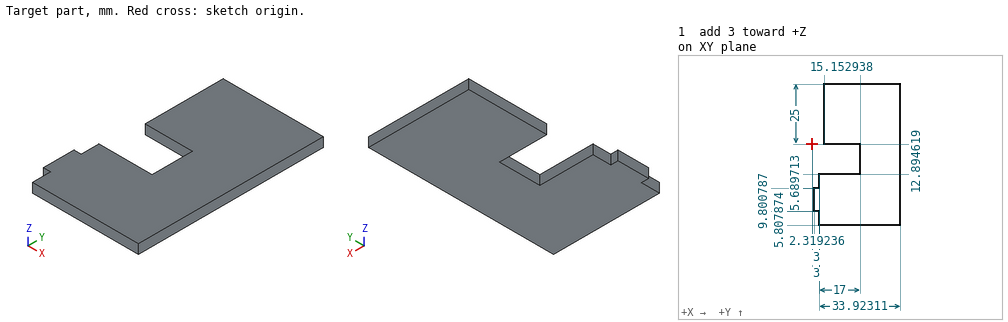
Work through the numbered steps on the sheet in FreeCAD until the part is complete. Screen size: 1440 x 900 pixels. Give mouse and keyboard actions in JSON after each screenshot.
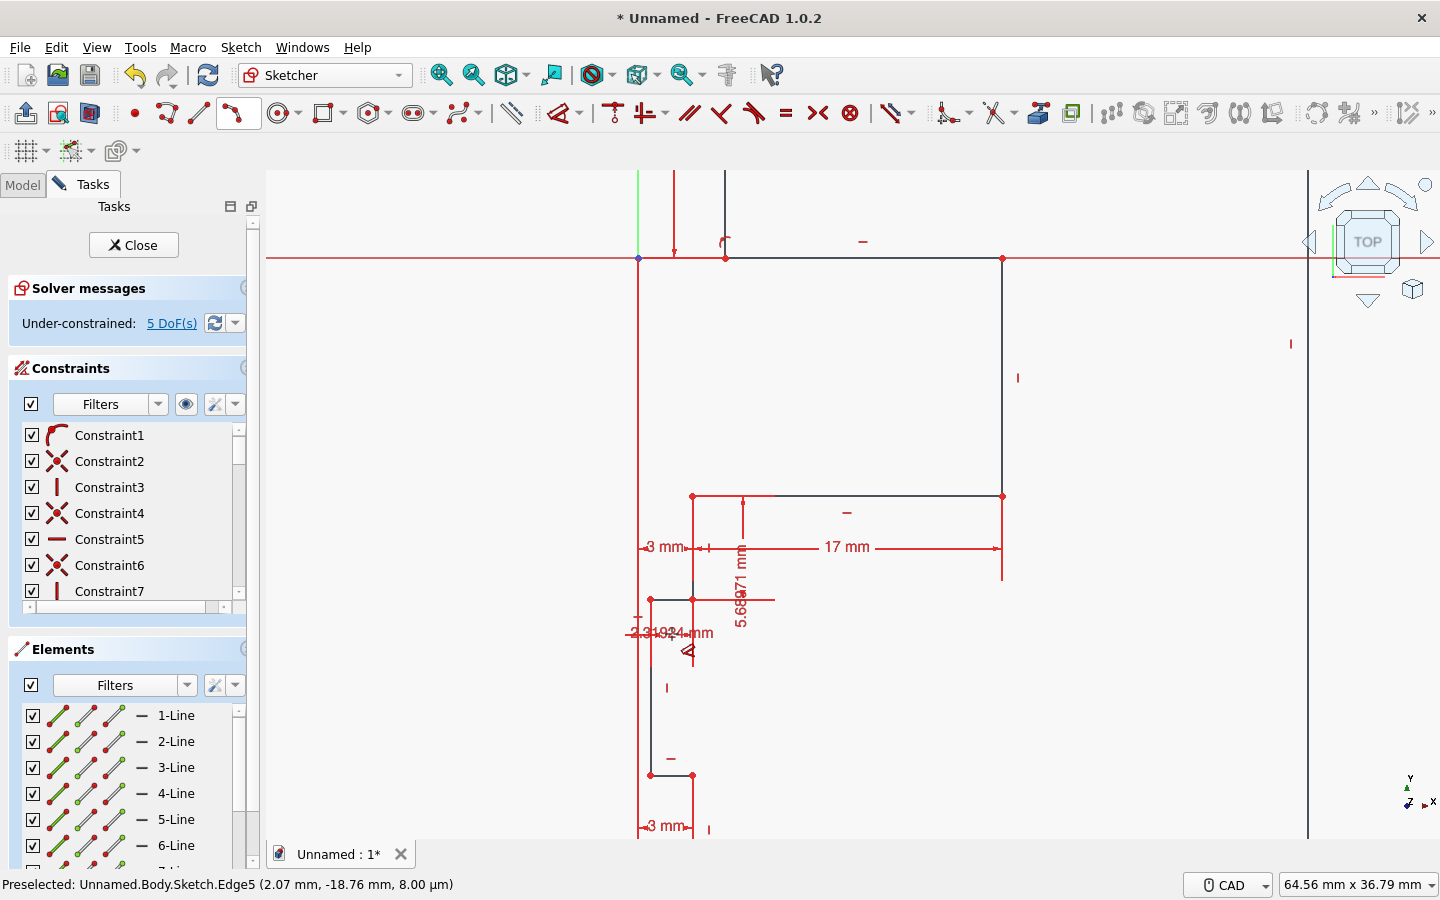
{"action": "left_click", "coordinate": [651, 652]}
{"action": "left_click", "coordinate": [617, 688]}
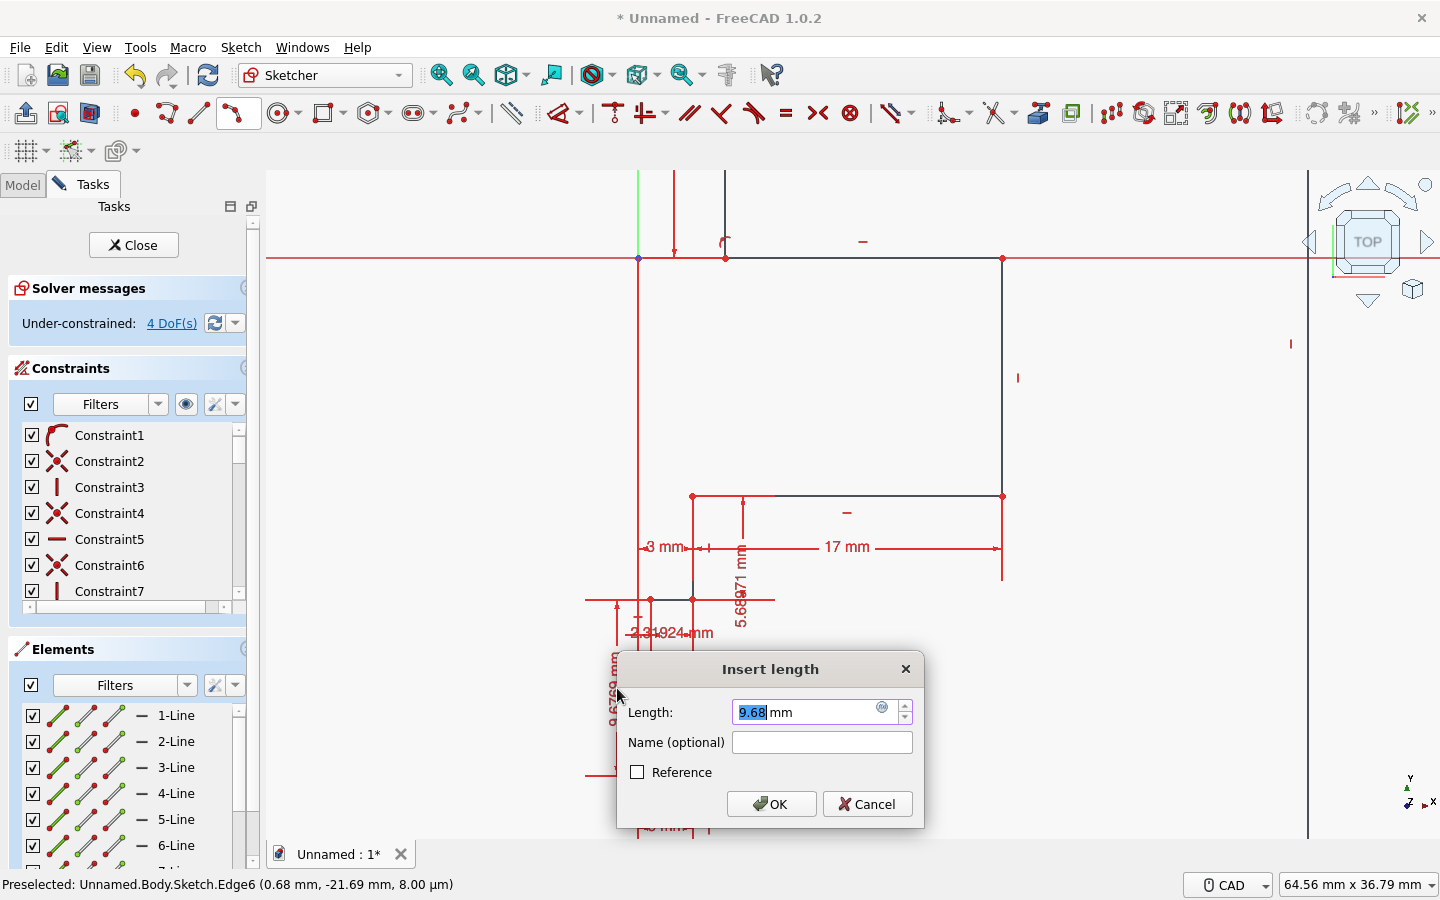
{"action": "type", "text": "9.800787"}
{"action": "key", "text": "Return"}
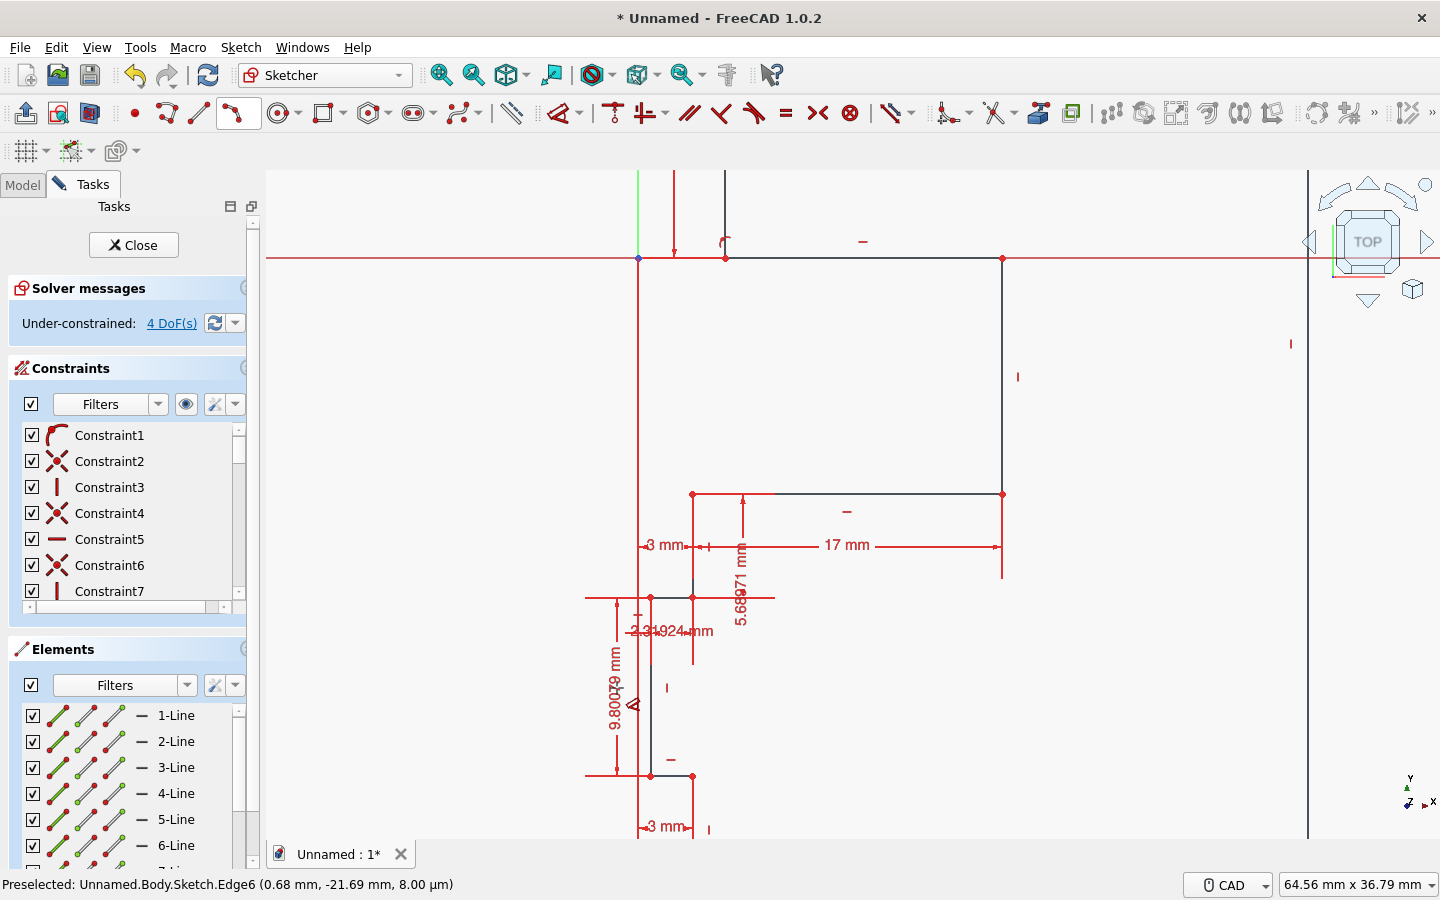
{"action": "left_click", "coordinate": [693, 808]}
{"action": "left_click", "coordinate": [659, 794]}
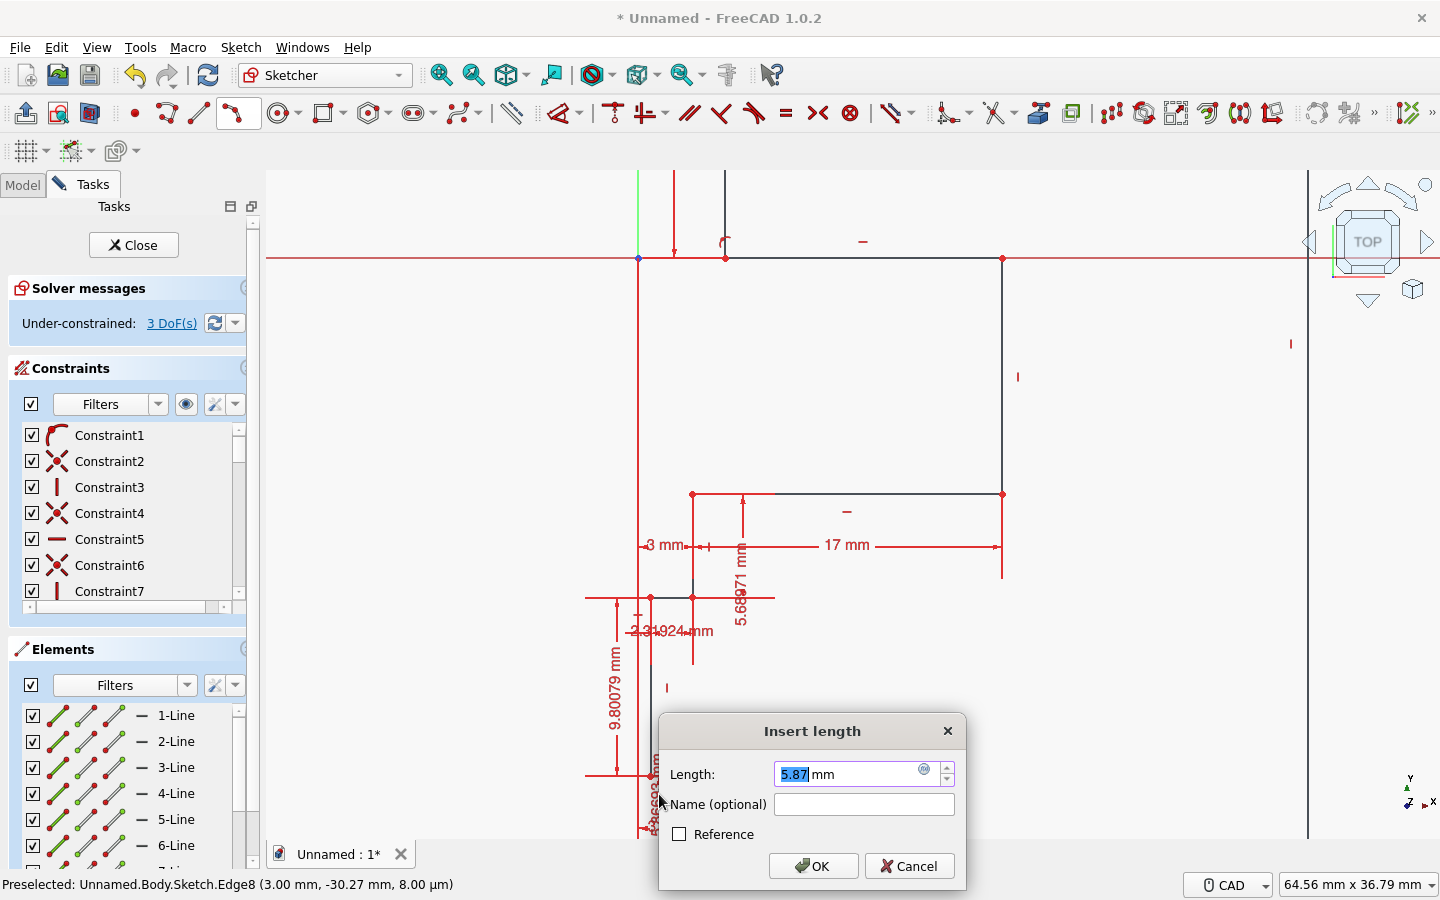
{"action": "type", "text": "5.807874"}
{"action": "key", "text": "Return"}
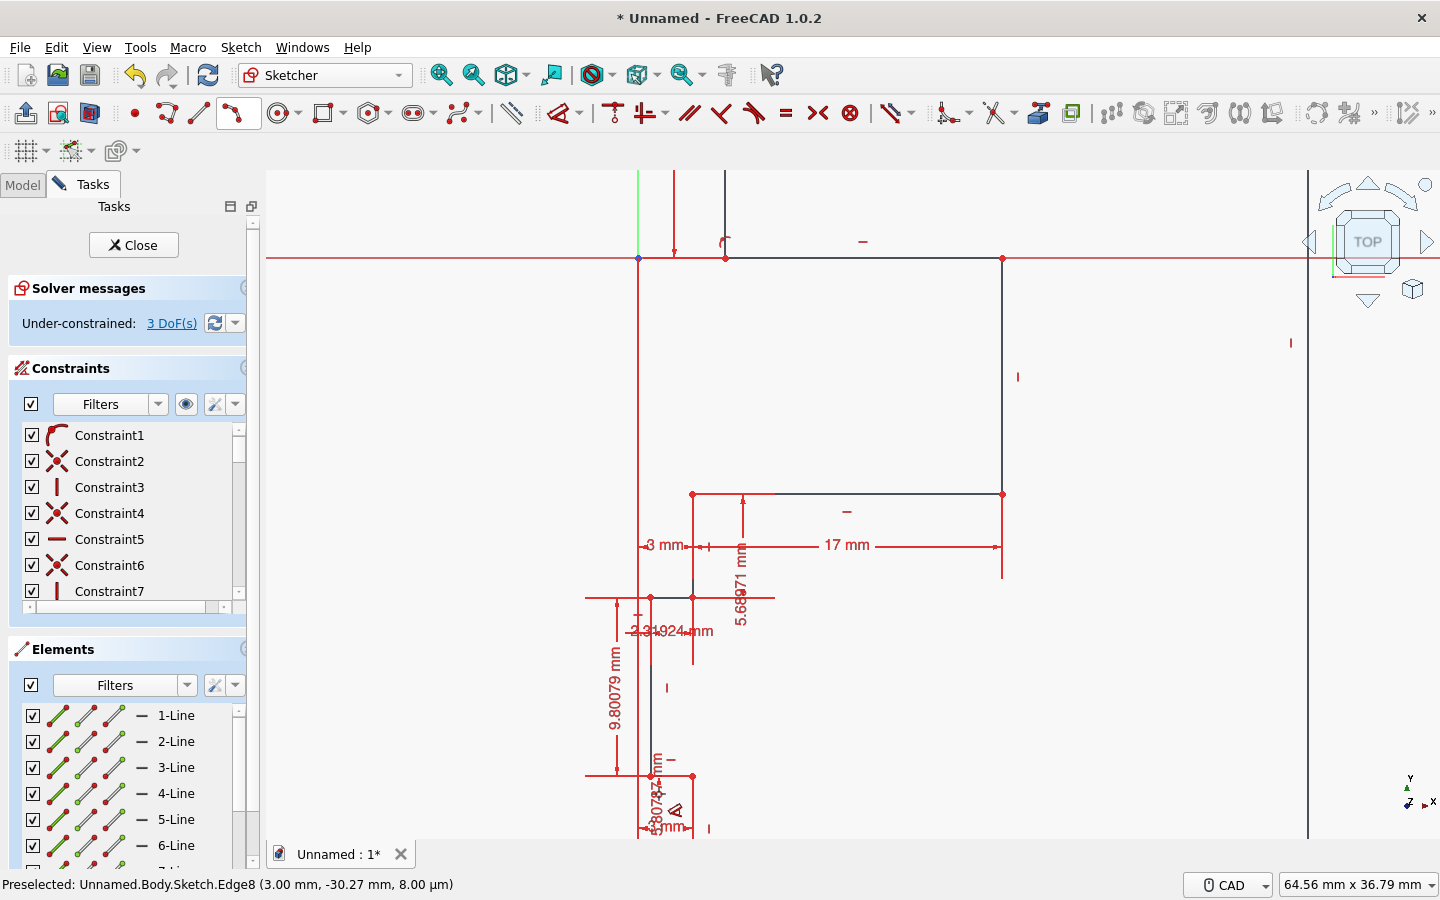
{"action": "scroll", "coordinate": [674, 599], "scroll_direction": "down", "scroll_amount": 5}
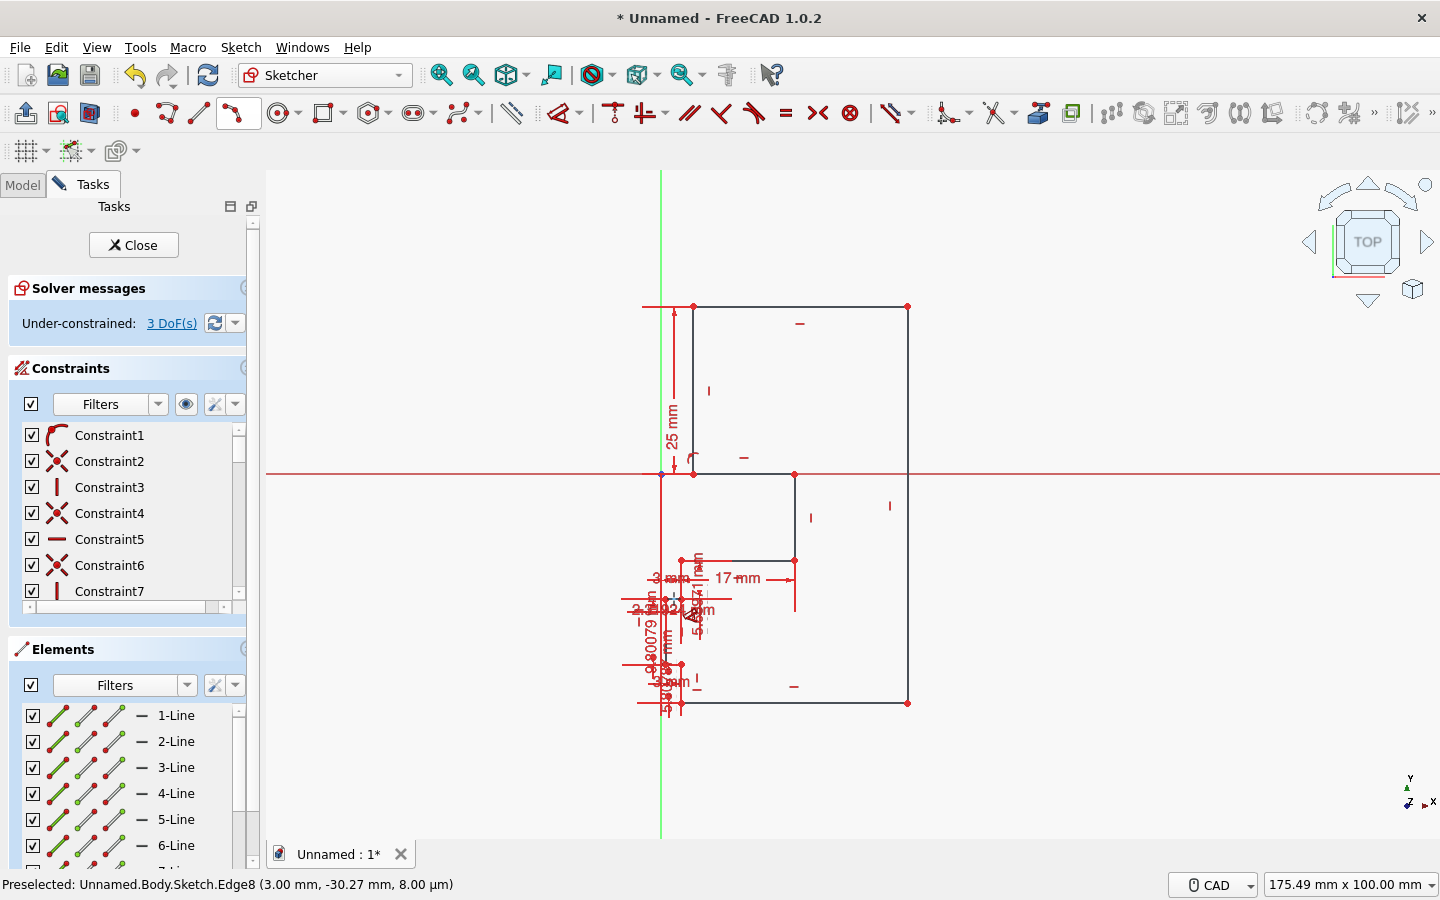
{"action": "left_click", "coordinate": [749, 703]}
{"action": "left_click", "coordinate": [794, 737]}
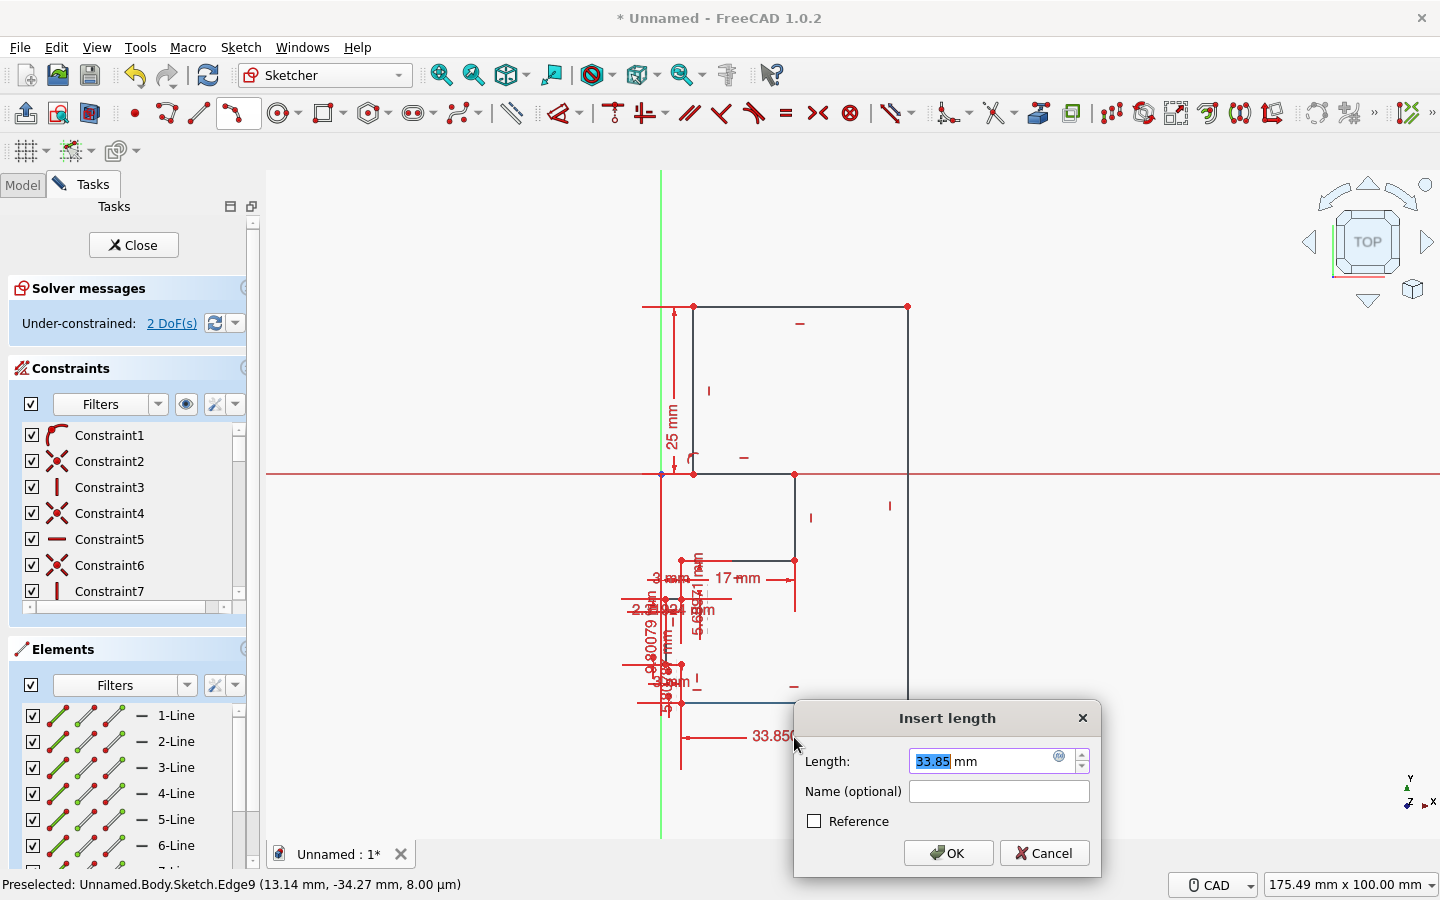
{"action": "type", "text": "33.92311"}
{"action": "key", "text": "Return"}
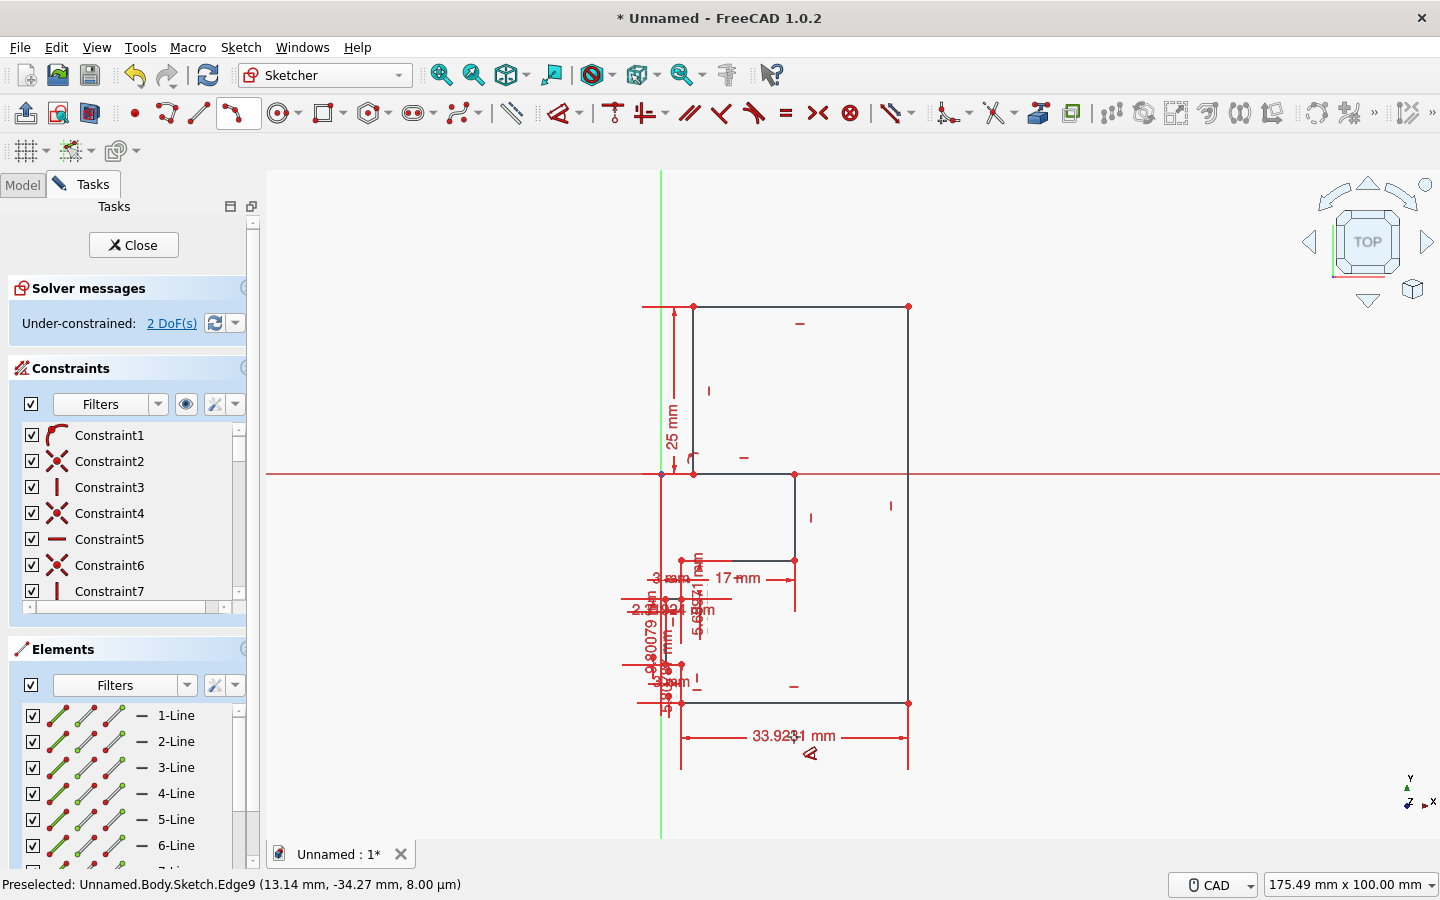
{"action": "left_click", "coordinate": [724, 474]}
{"action": "left_click", "coordinate": [767, 440]}